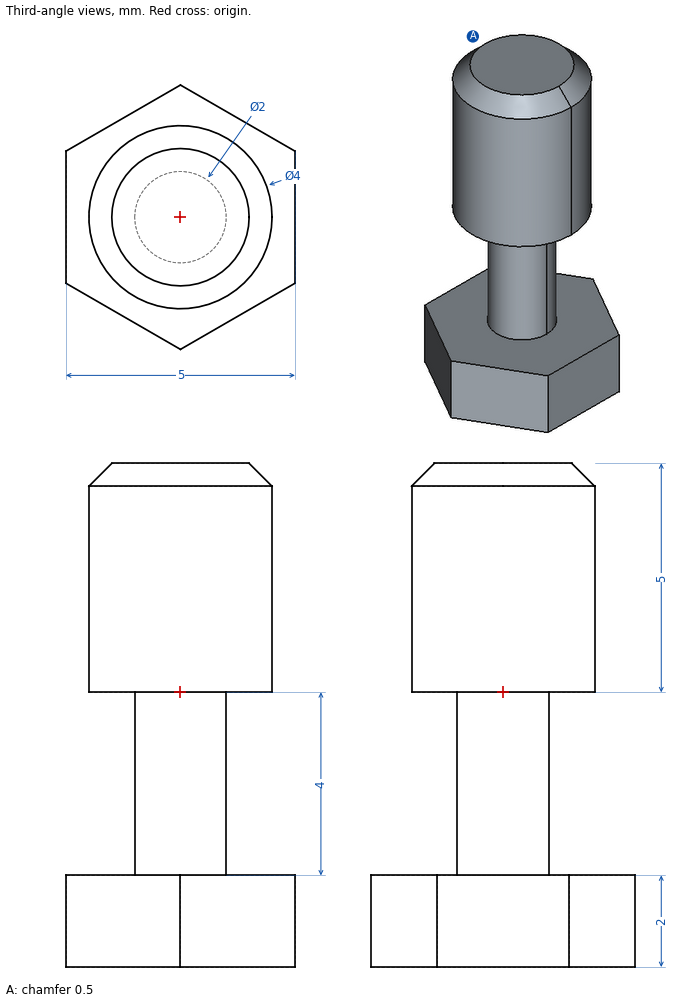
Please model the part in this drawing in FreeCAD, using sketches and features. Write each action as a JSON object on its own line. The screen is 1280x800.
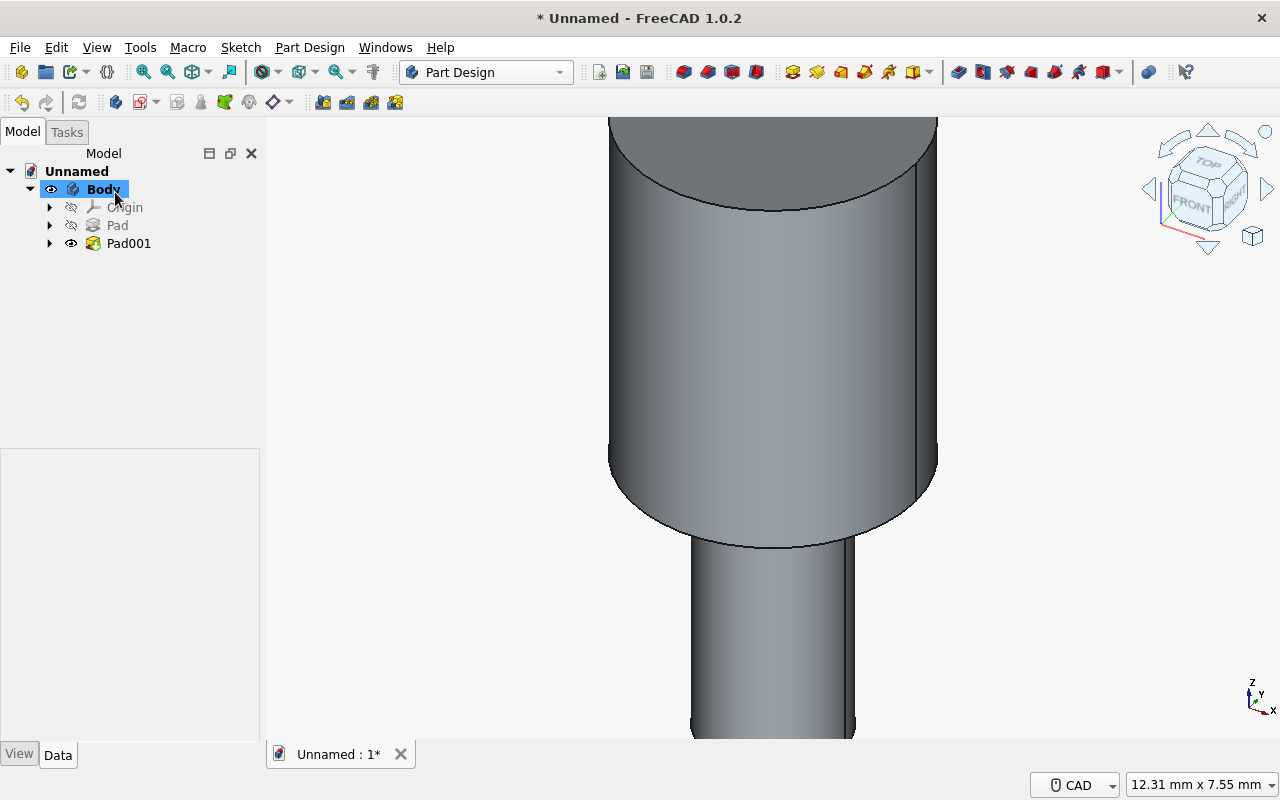
{"action": "left_click", "coordinate": [144, 72]}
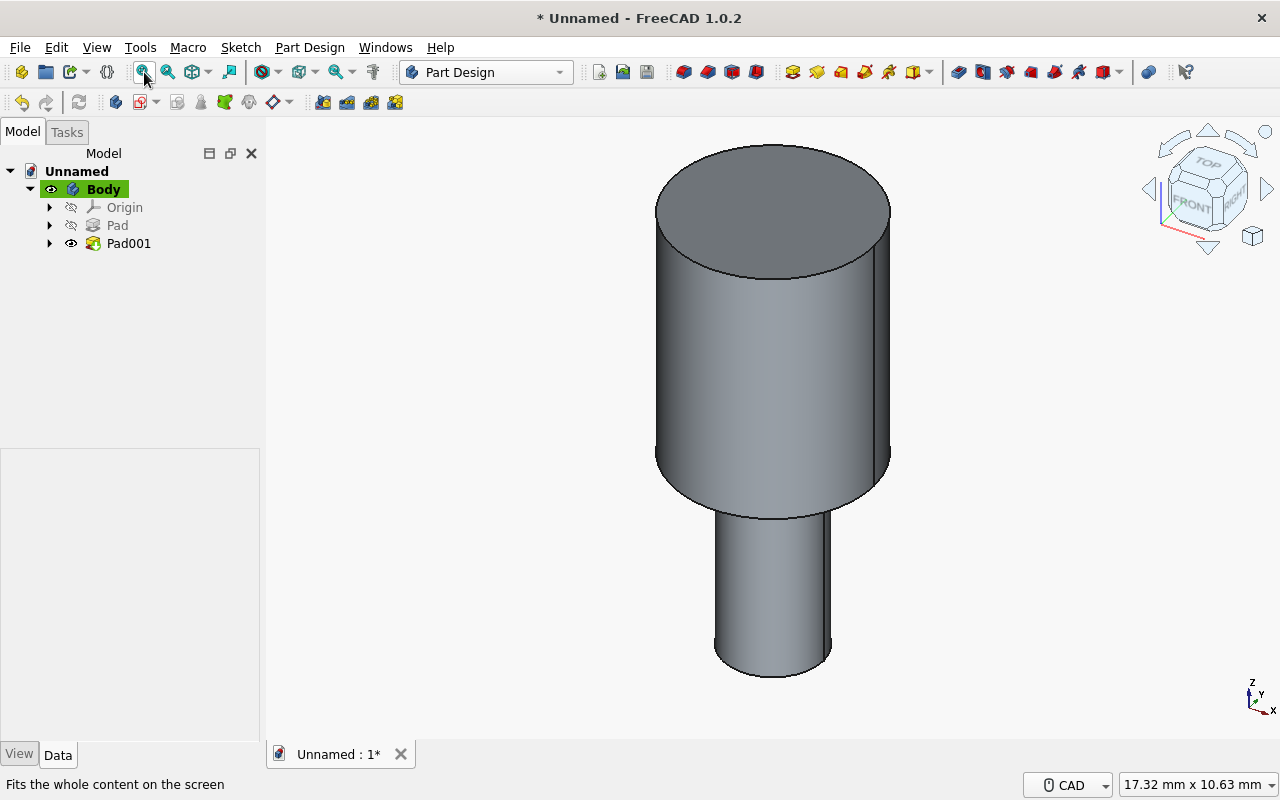
{"action": "key", "text": "5"}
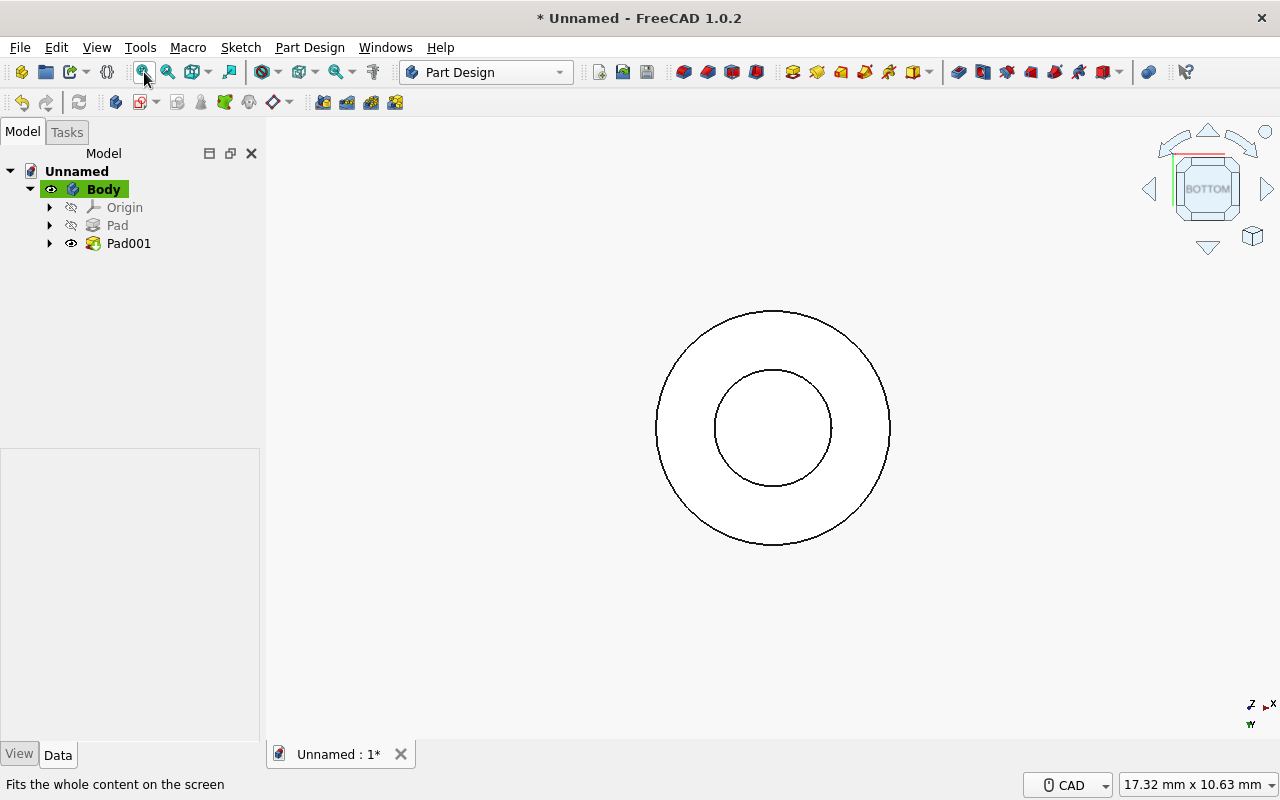
{"action": "left_click", "coordinate": [144, 72]}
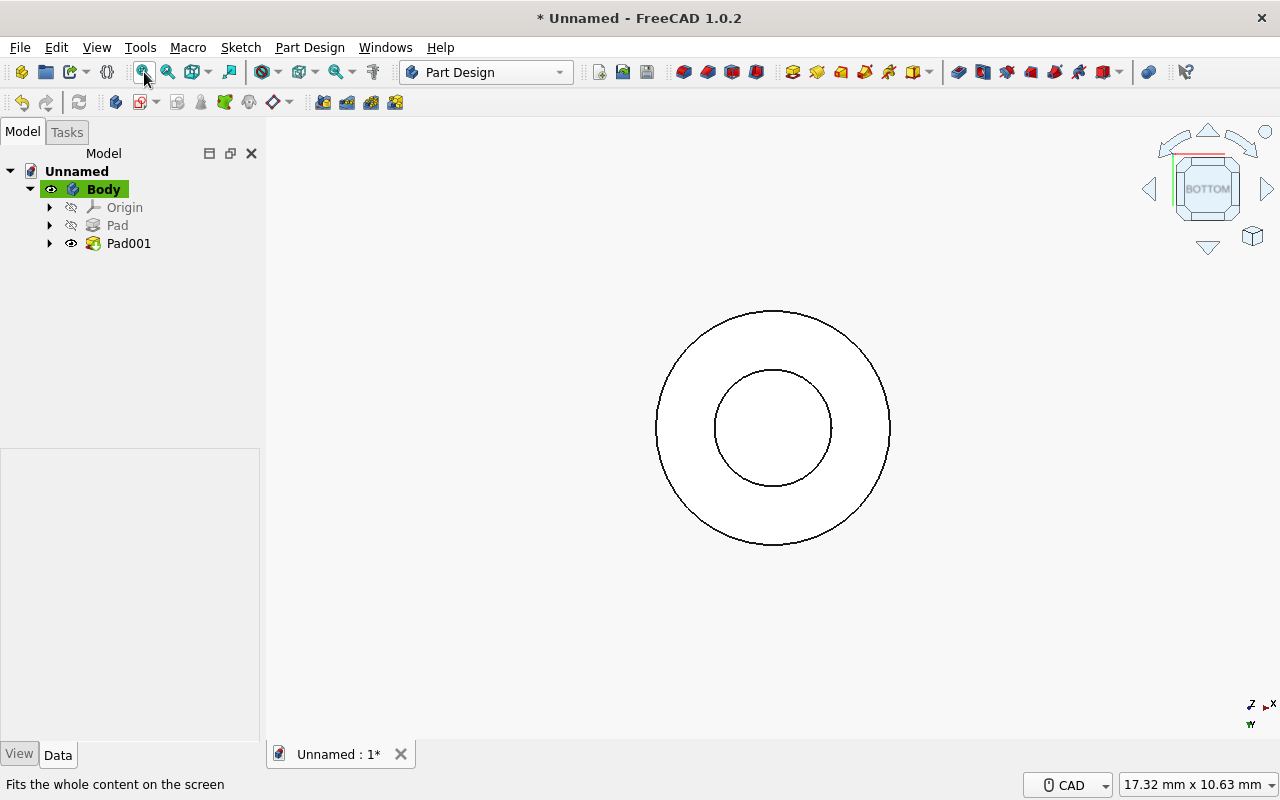
{"action": "left_click", "coordinate": [773, 427]}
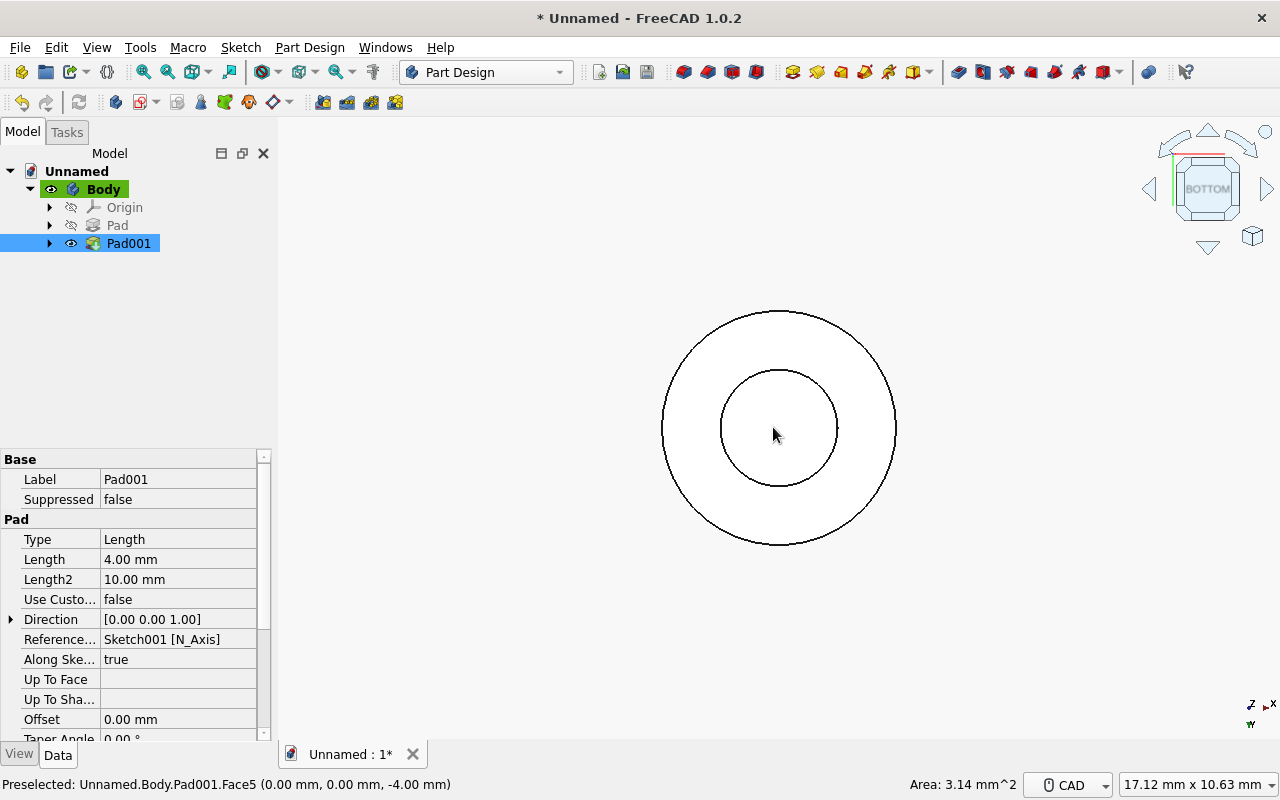
{"action": "left_click", "coordinate": [140, 102]}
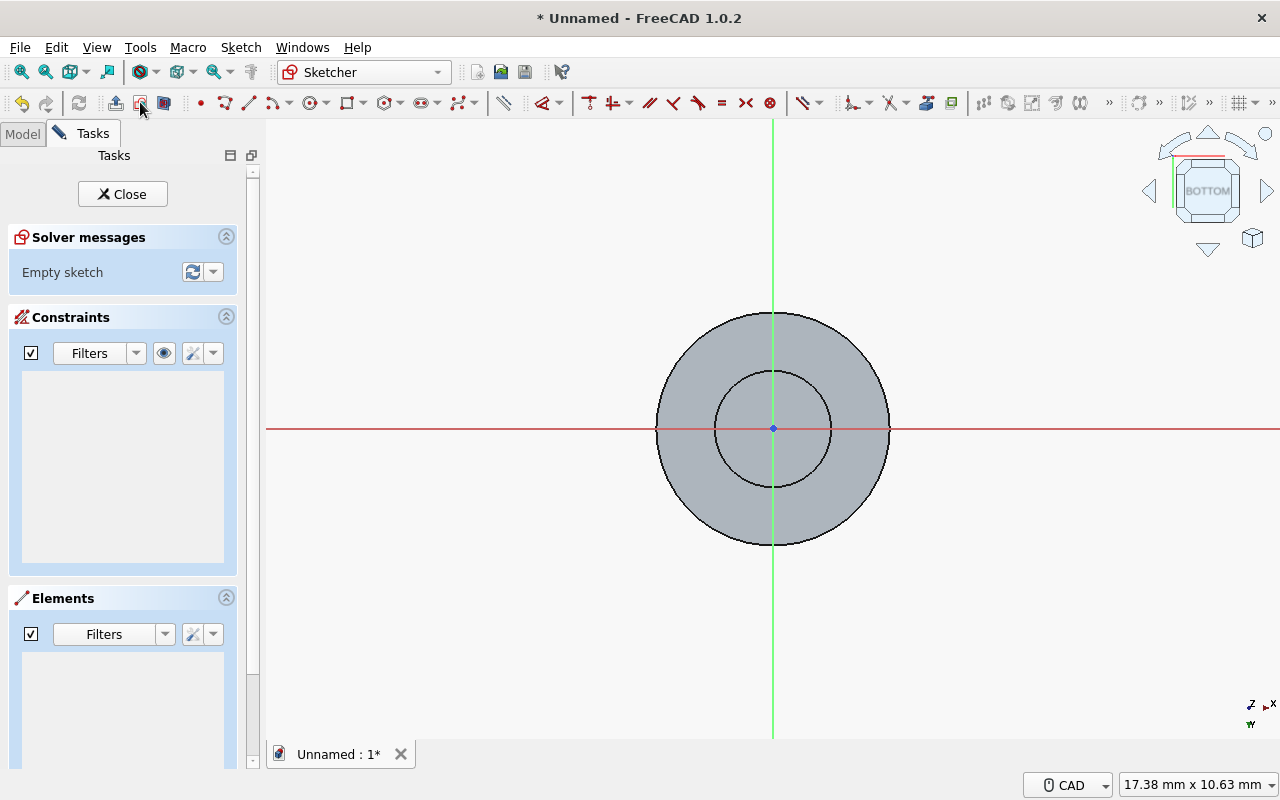
{"action": "left_click", "coordinate": [384, 104]}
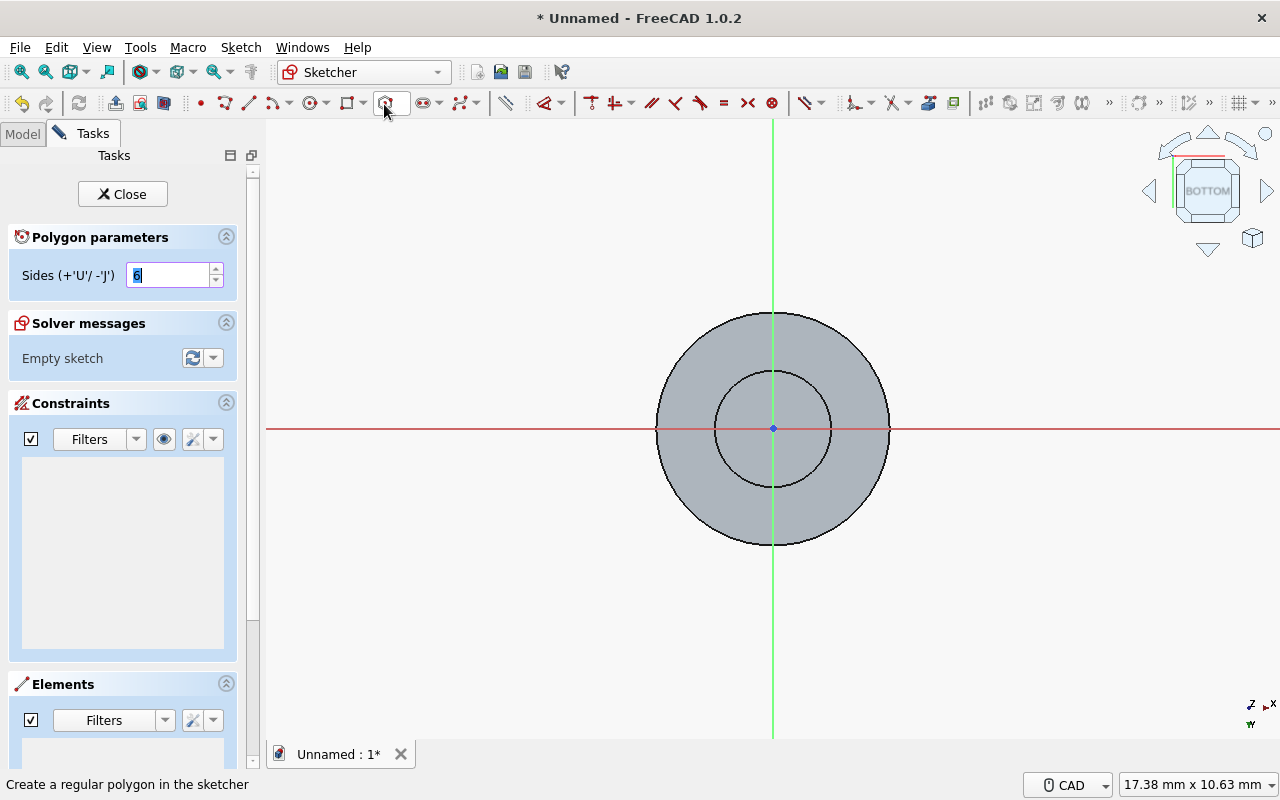
{"action": "left_click", "coordinate": [773, 429]}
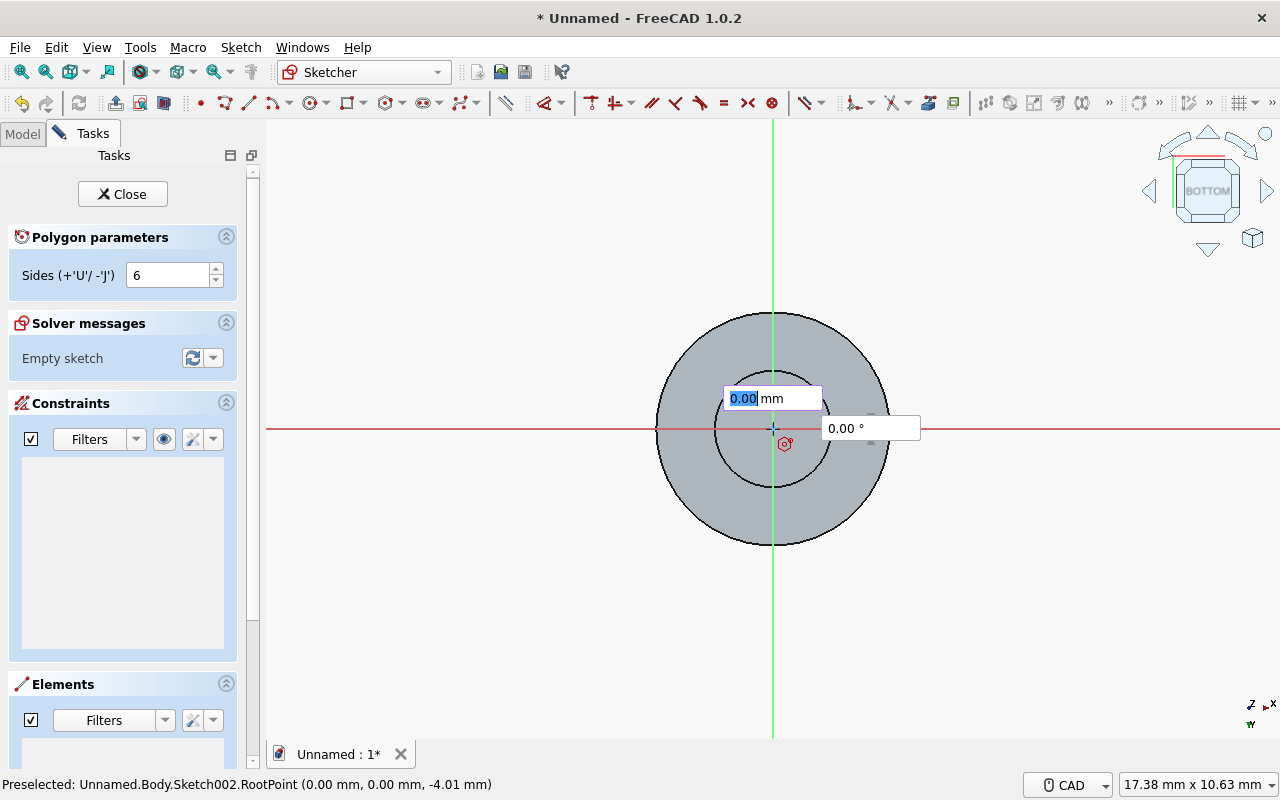
{"action": "left_click", "coordinate": [773, 597]}
{"action": "right_click", "coordinate": [773, 597]}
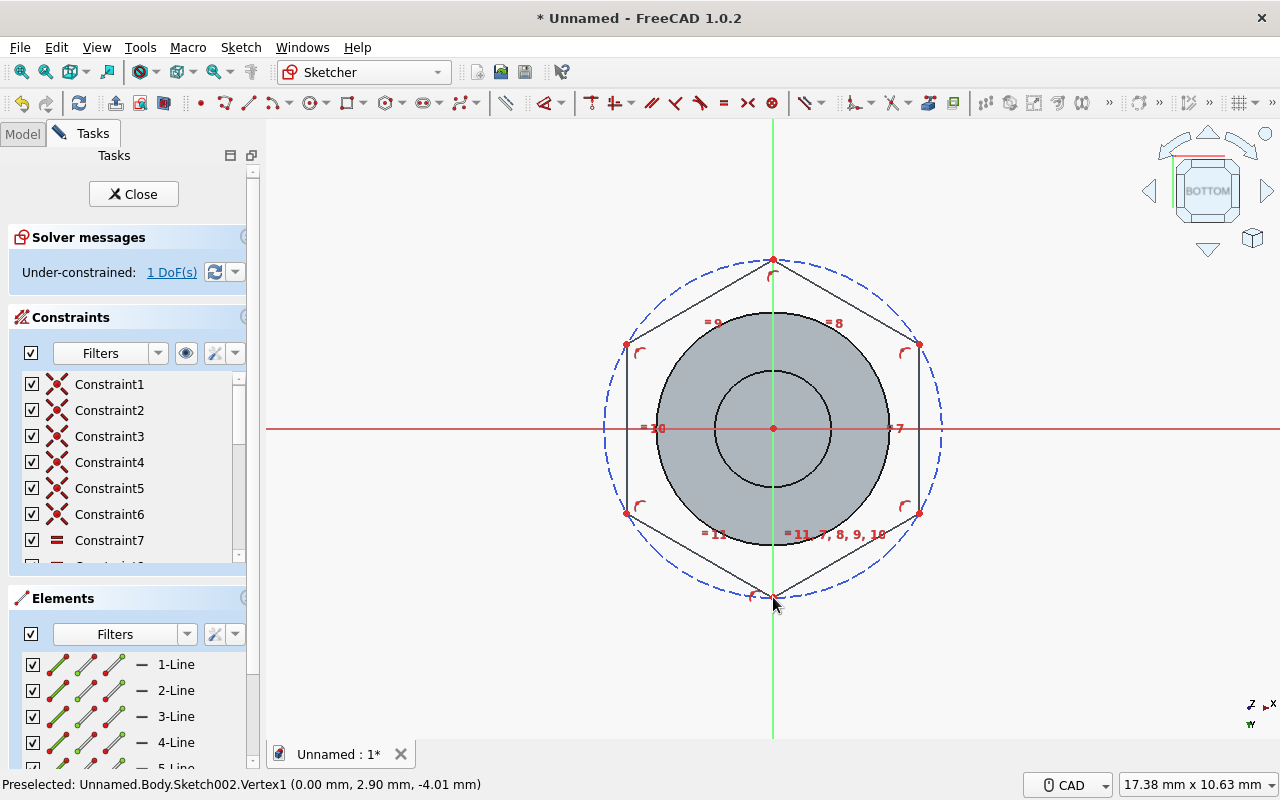
{"action": "key", "text": "d"}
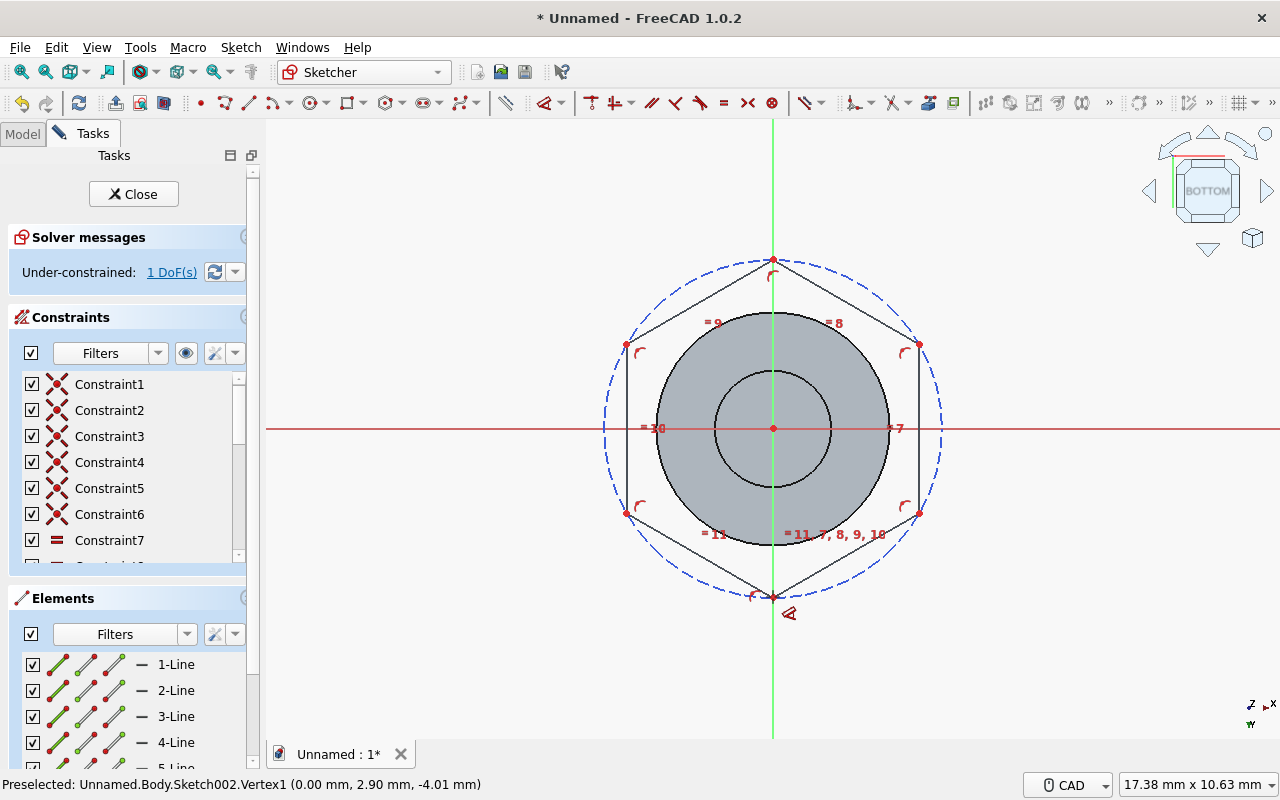
{"action": "left_click", "coordinate": [627, 345]}